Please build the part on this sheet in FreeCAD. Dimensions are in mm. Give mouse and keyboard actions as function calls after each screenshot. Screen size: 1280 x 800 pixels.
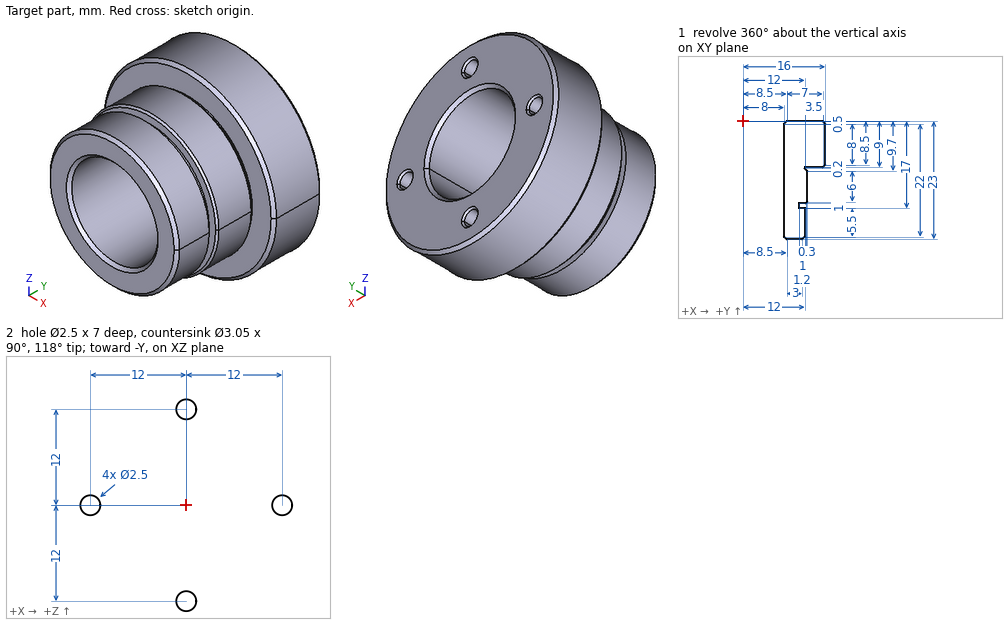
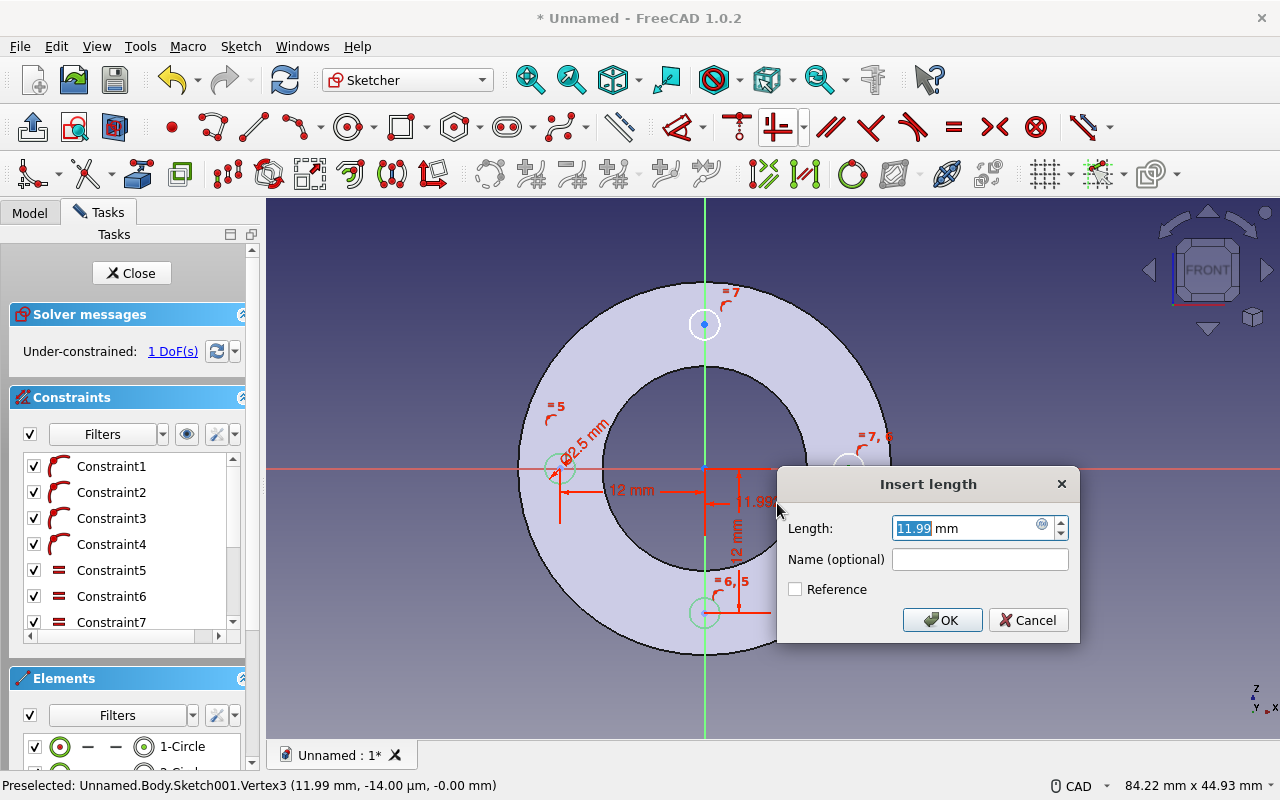
text(12)
key(Return)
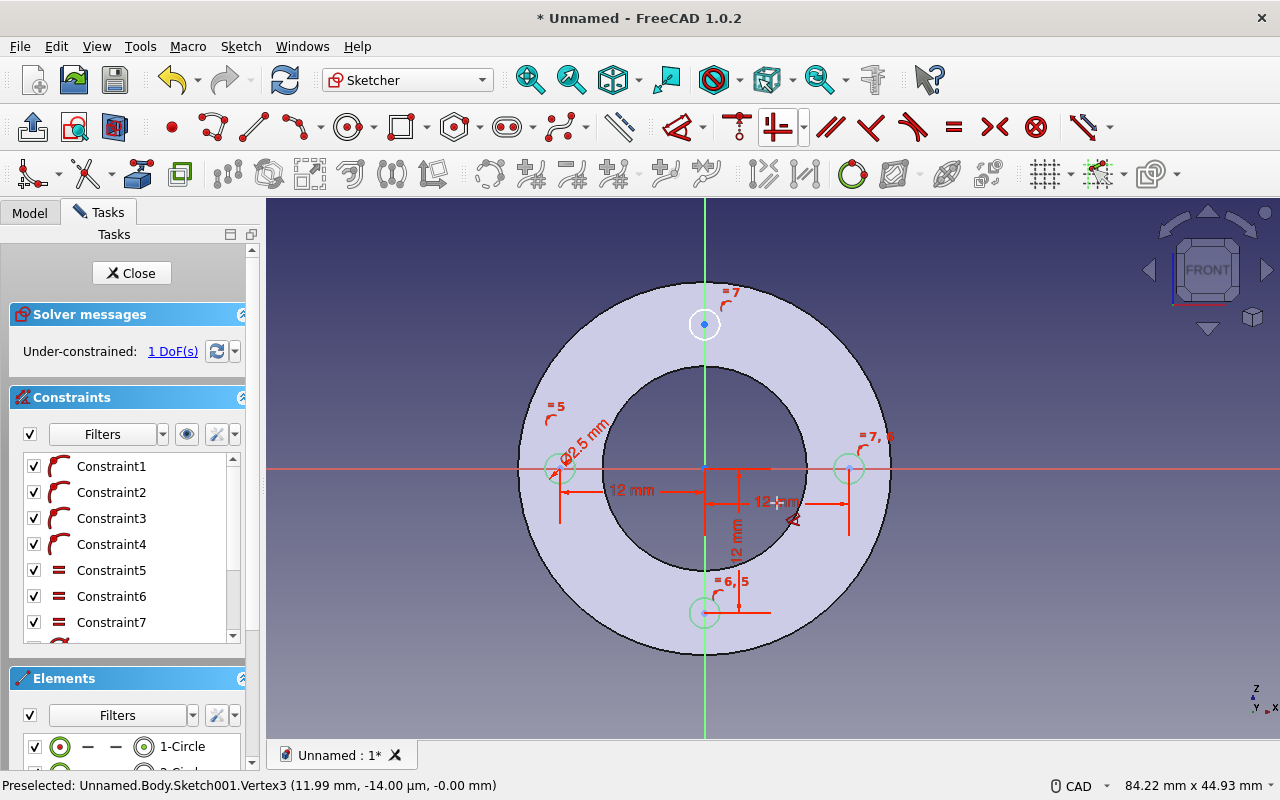
click(705, 325)
click(739, 397)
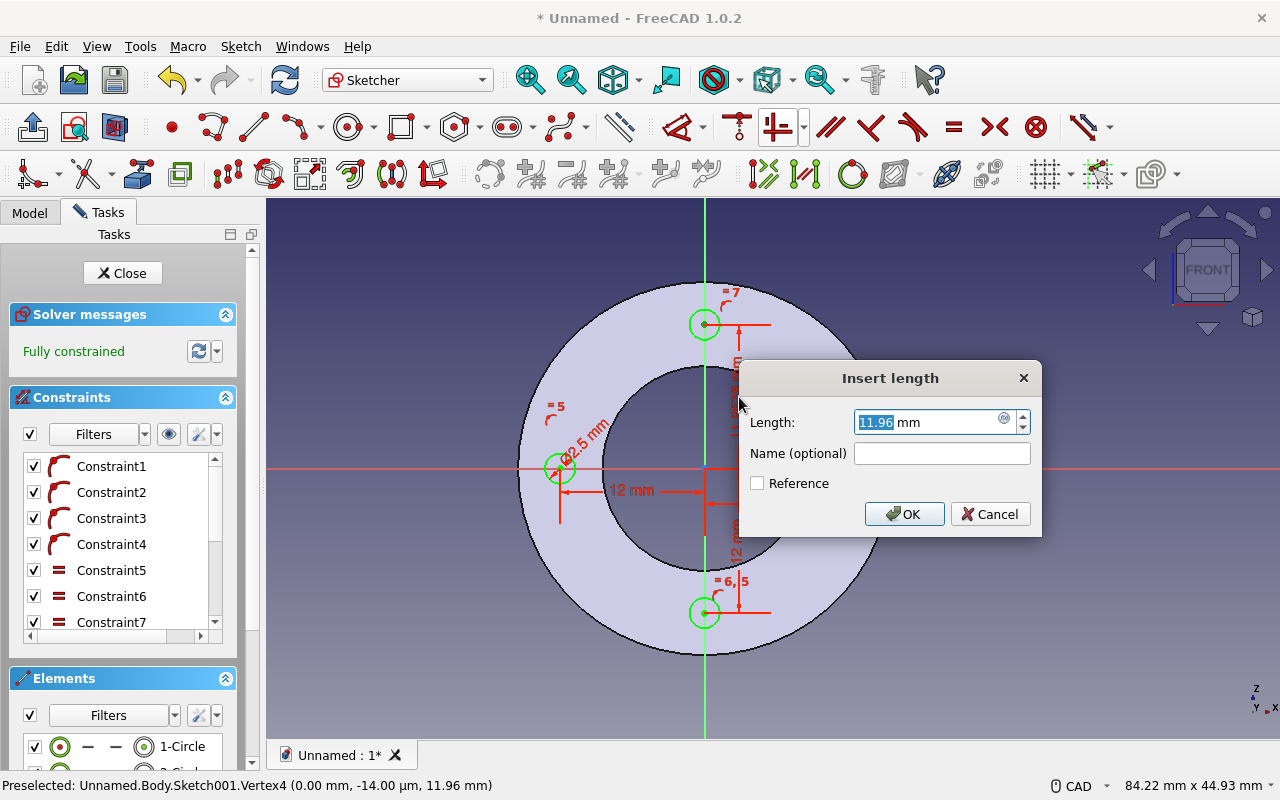
text(12)
key(Return)
key(Escape)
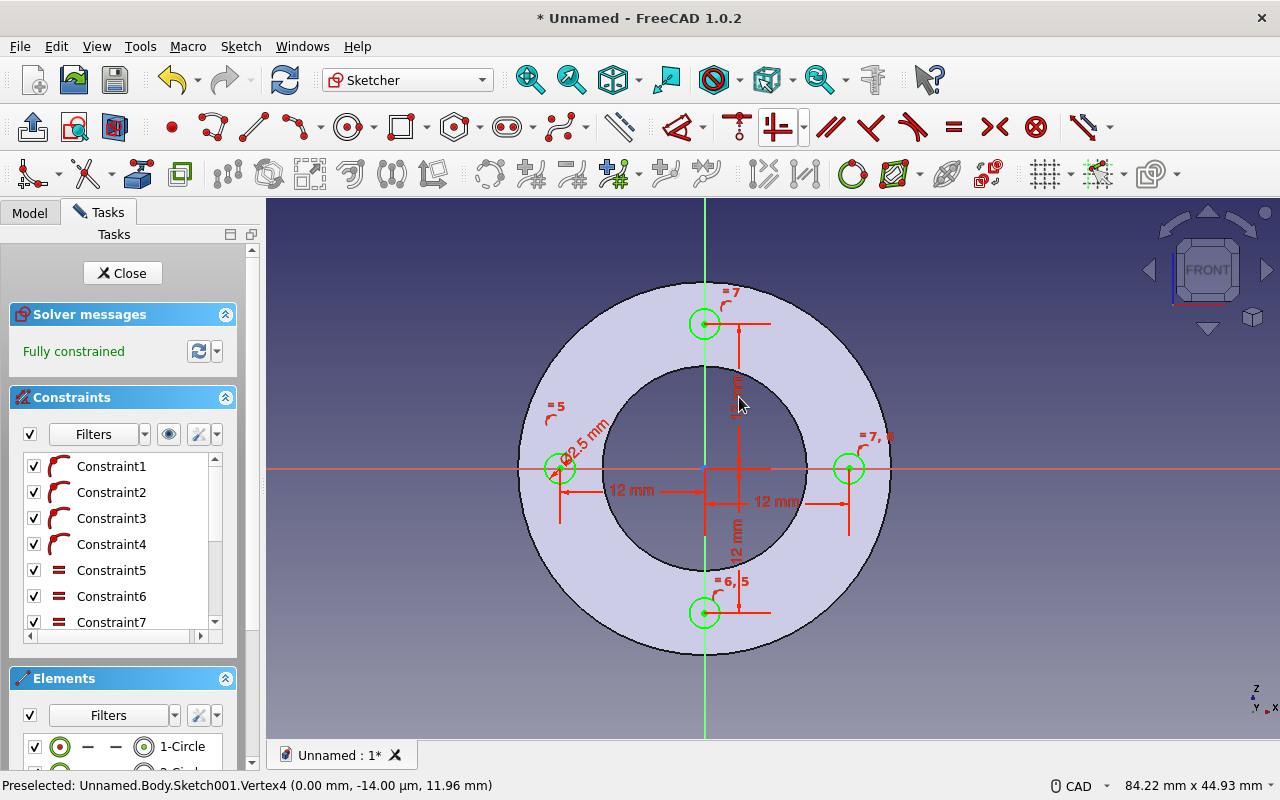
click(123, 273)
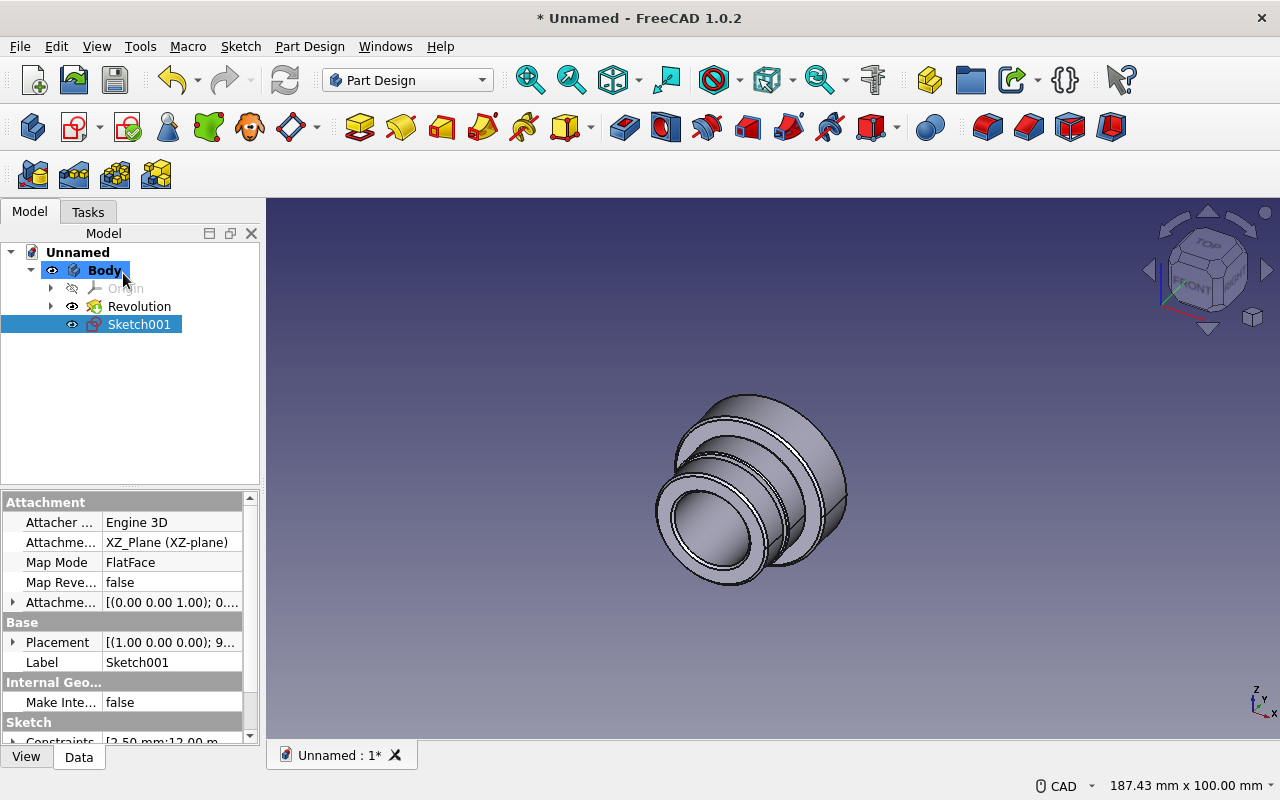
click(666, 128)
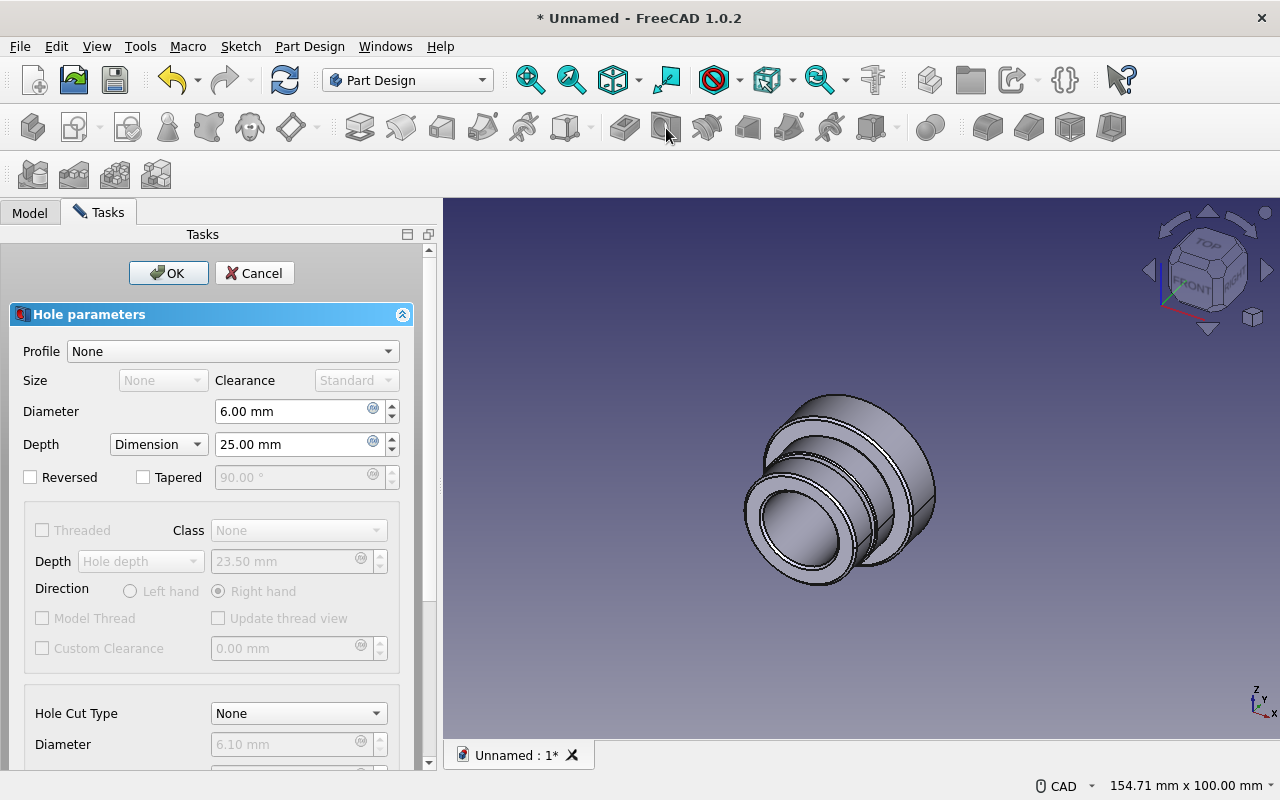
triple_click(300, 412)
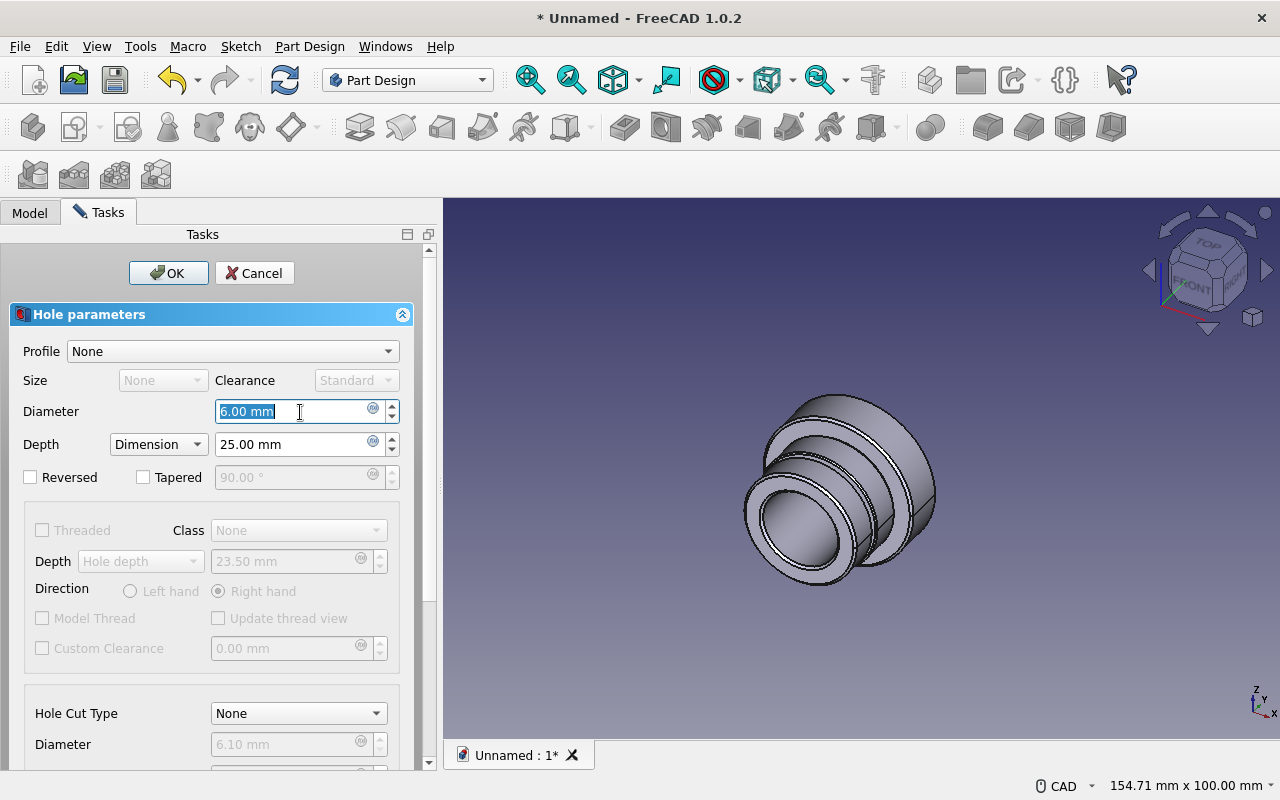
text(2.5)
key(Tab)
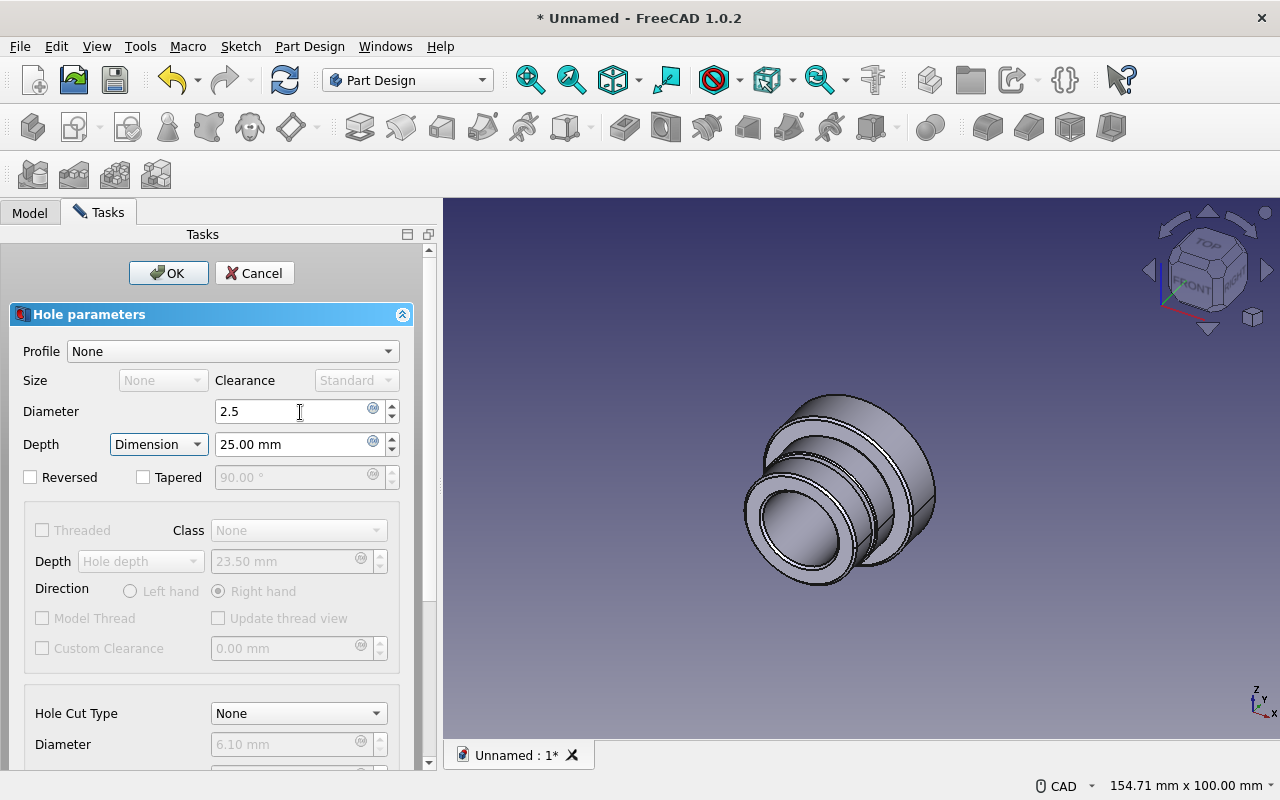
triple_click(300, 444)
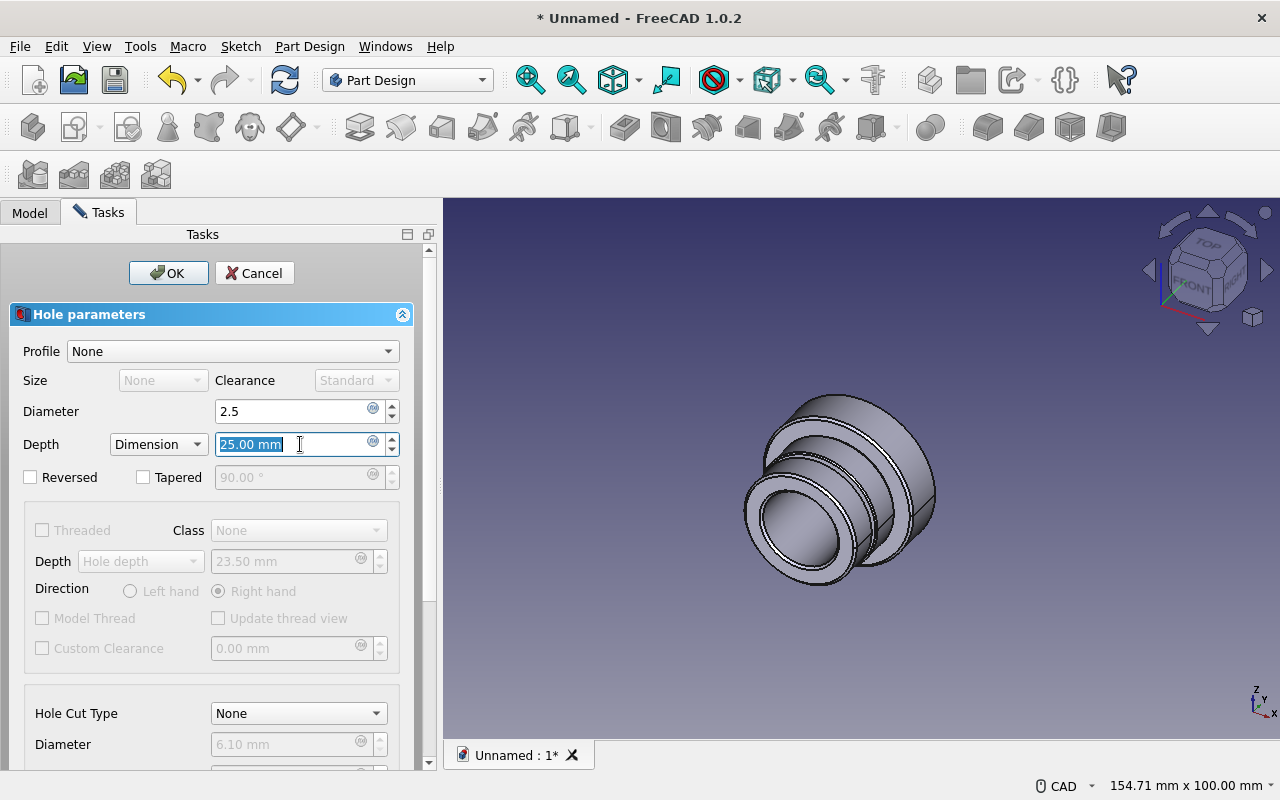
text(7)
key(Tab)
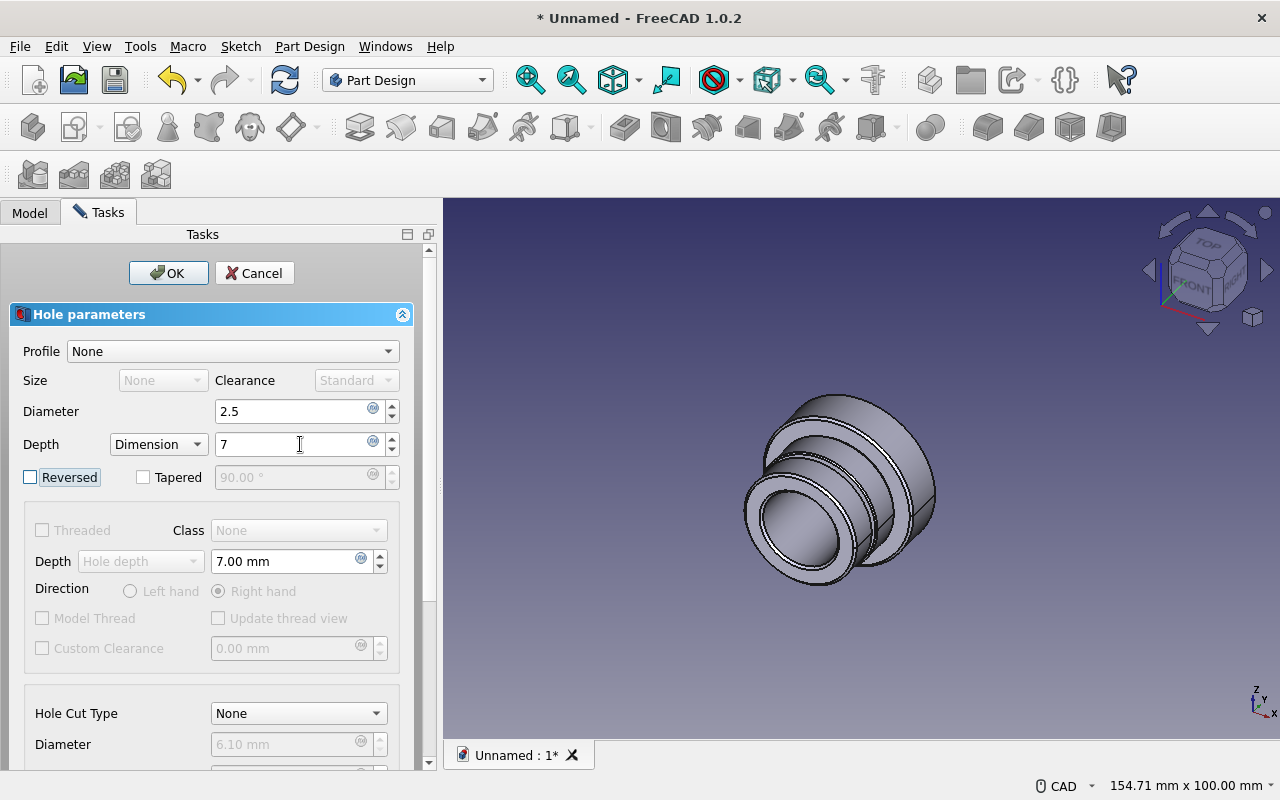
click(31, 477)